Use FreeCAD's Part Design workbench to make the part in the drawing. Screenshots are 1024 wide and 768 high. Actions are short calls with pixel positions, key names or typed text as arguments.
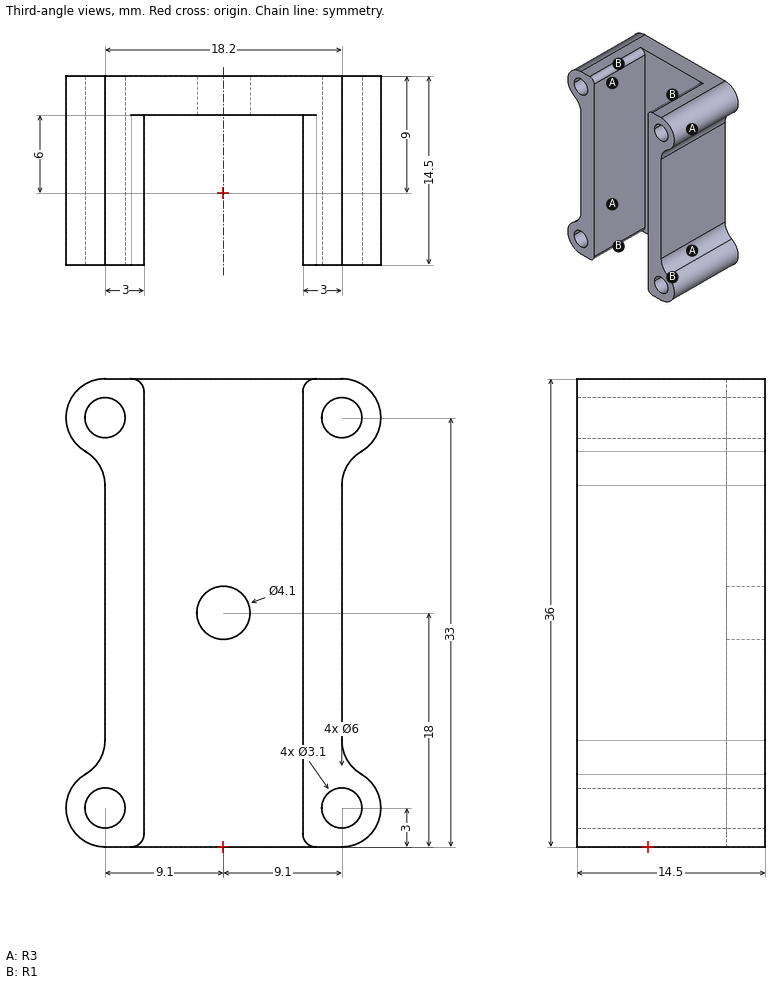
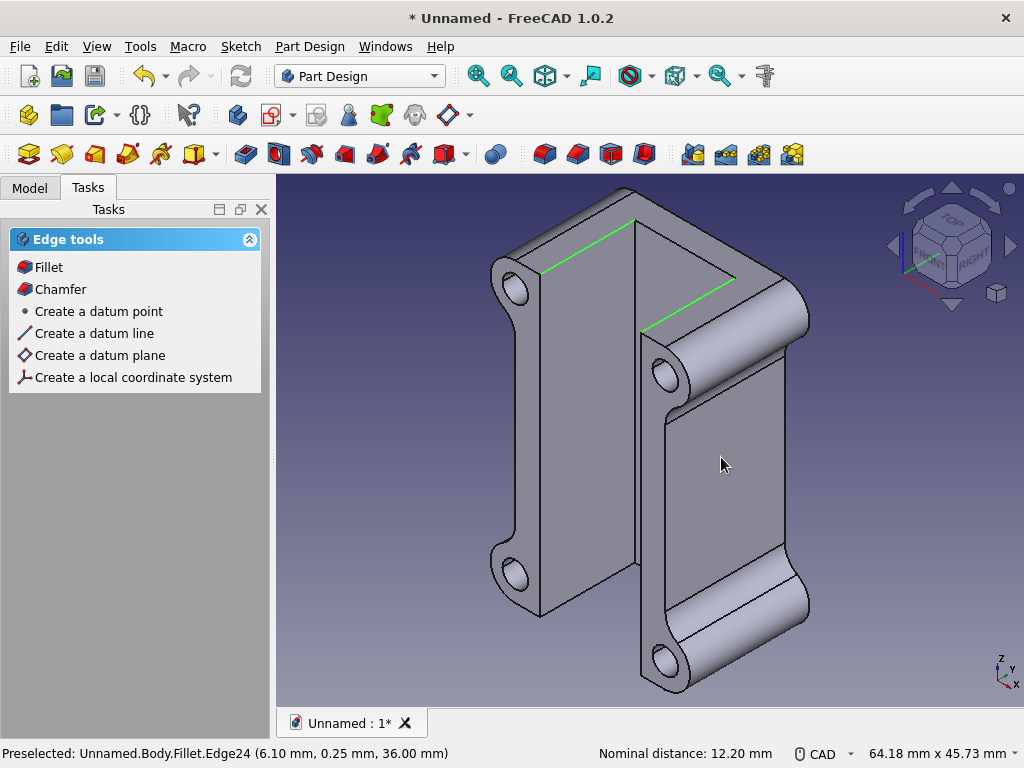
key(1)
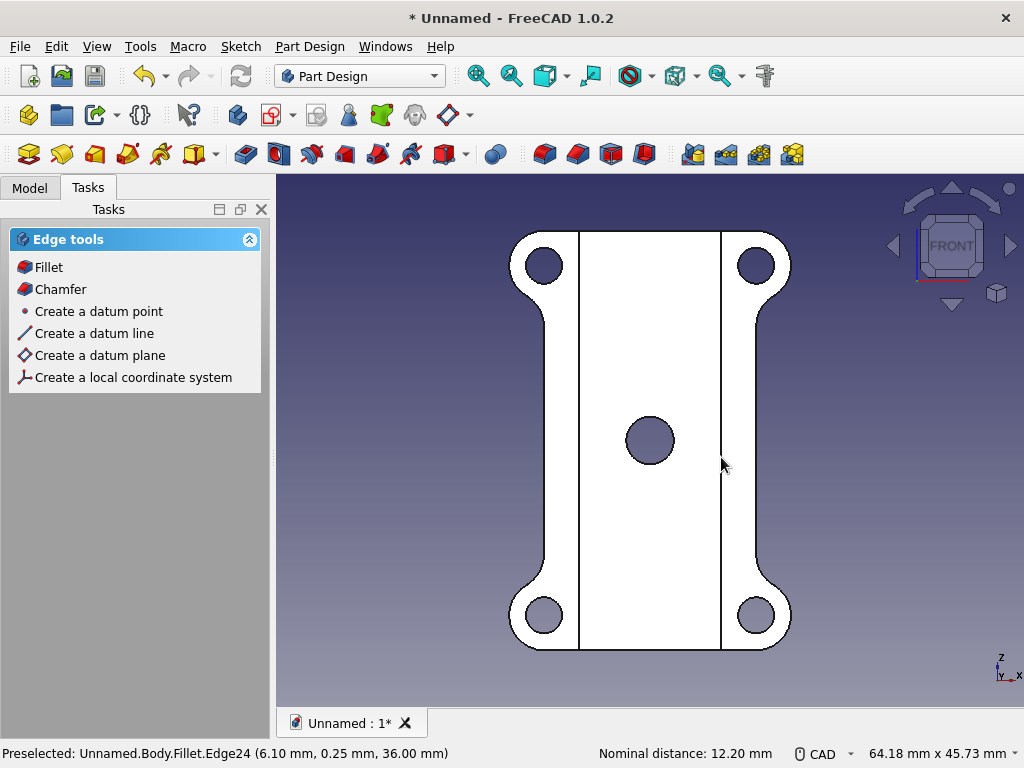
key(3)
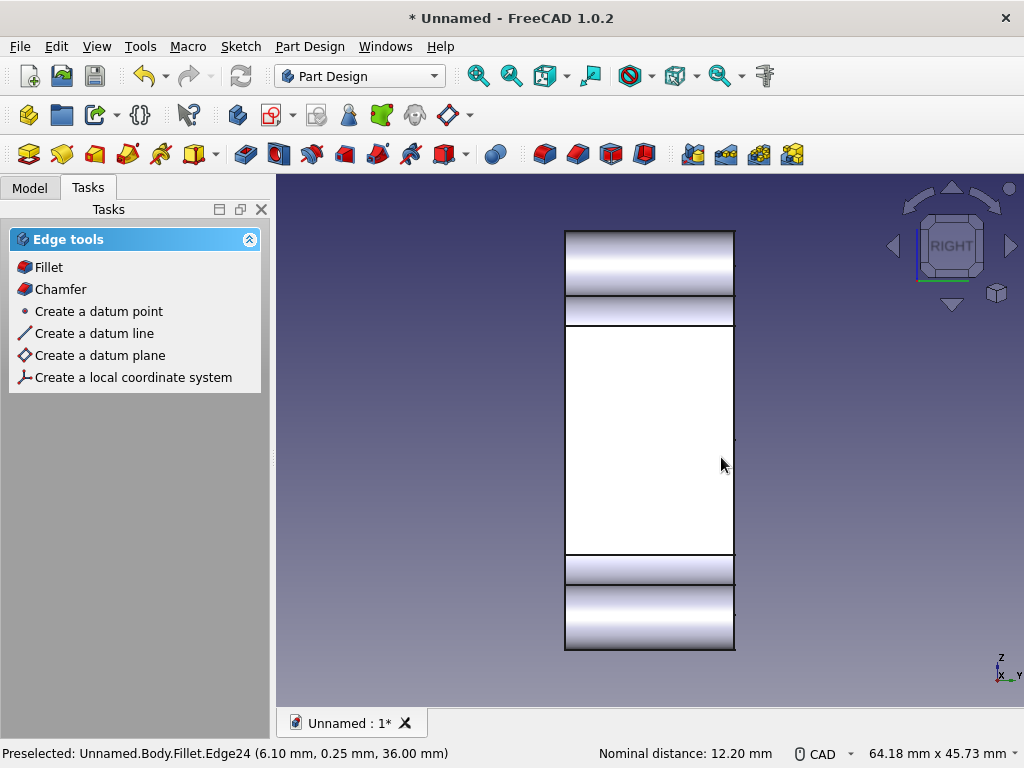
key(5)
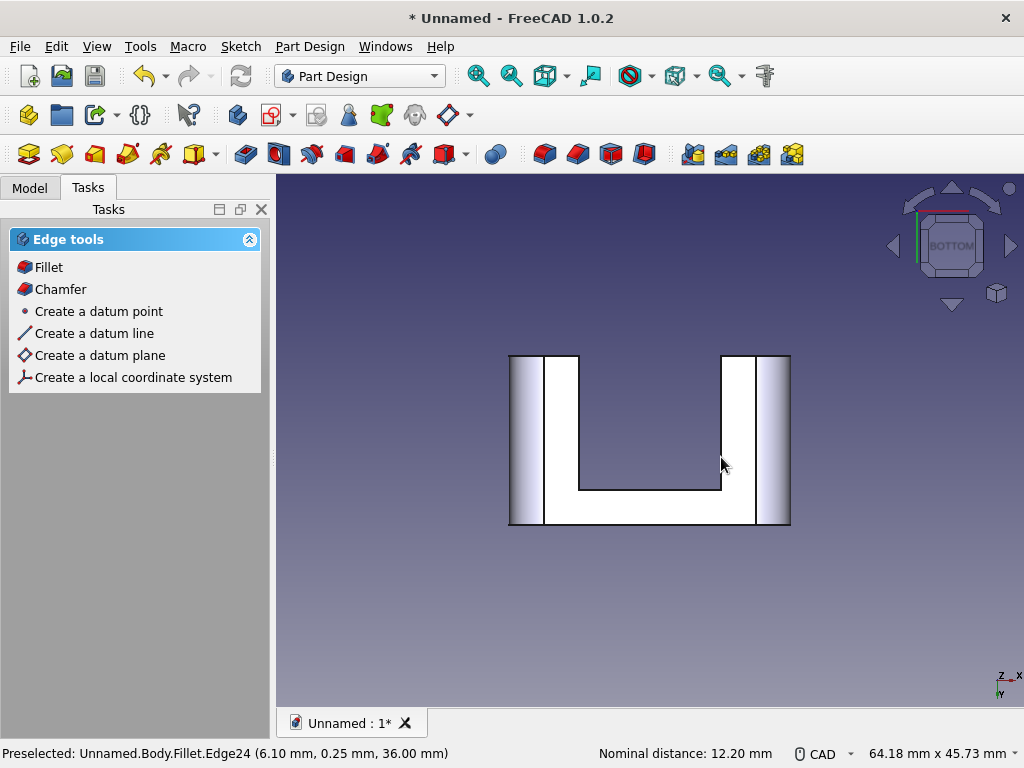
click(479, 76)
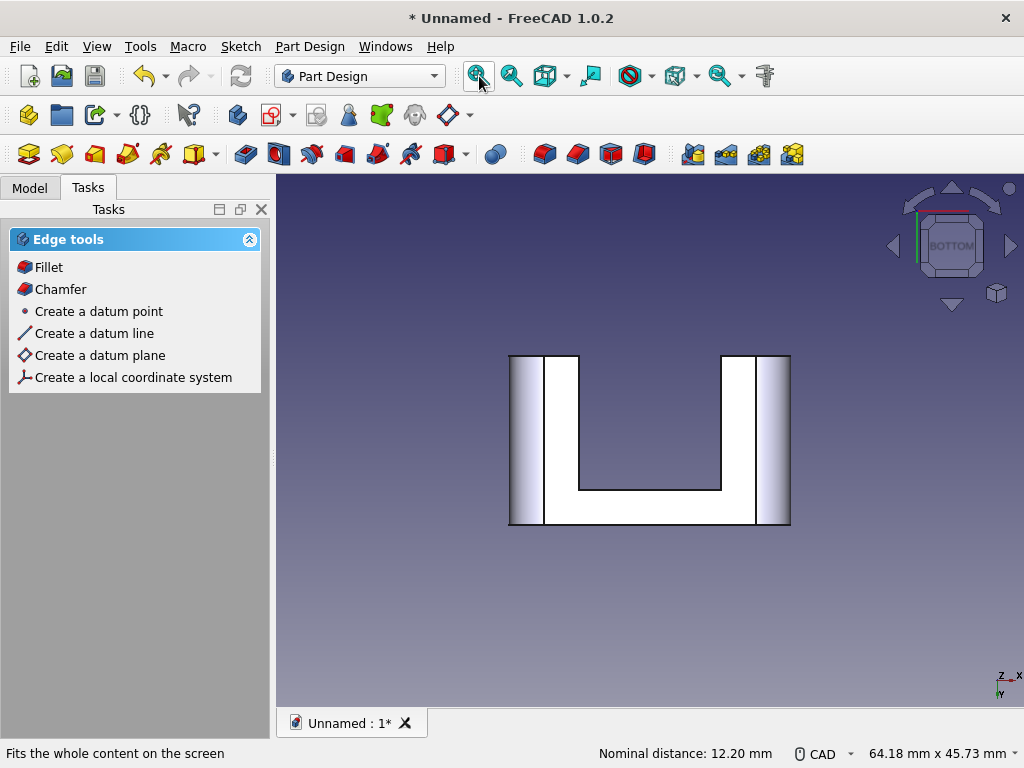
click(721, 422, ctrl)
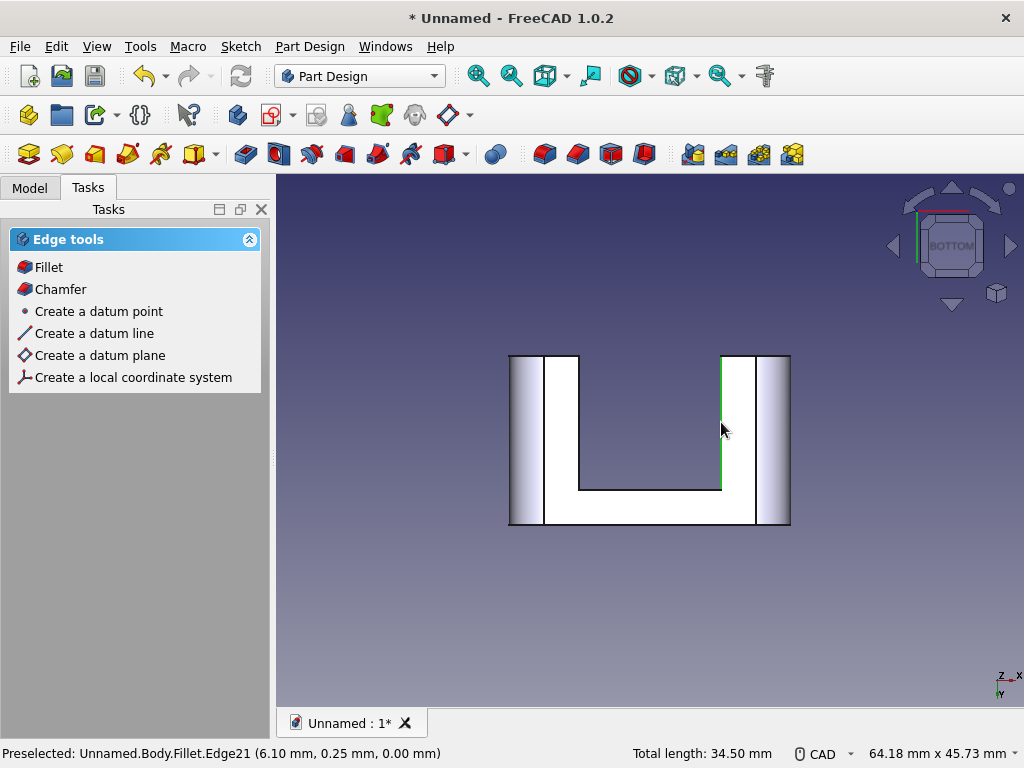
click(579, 422, ctrl)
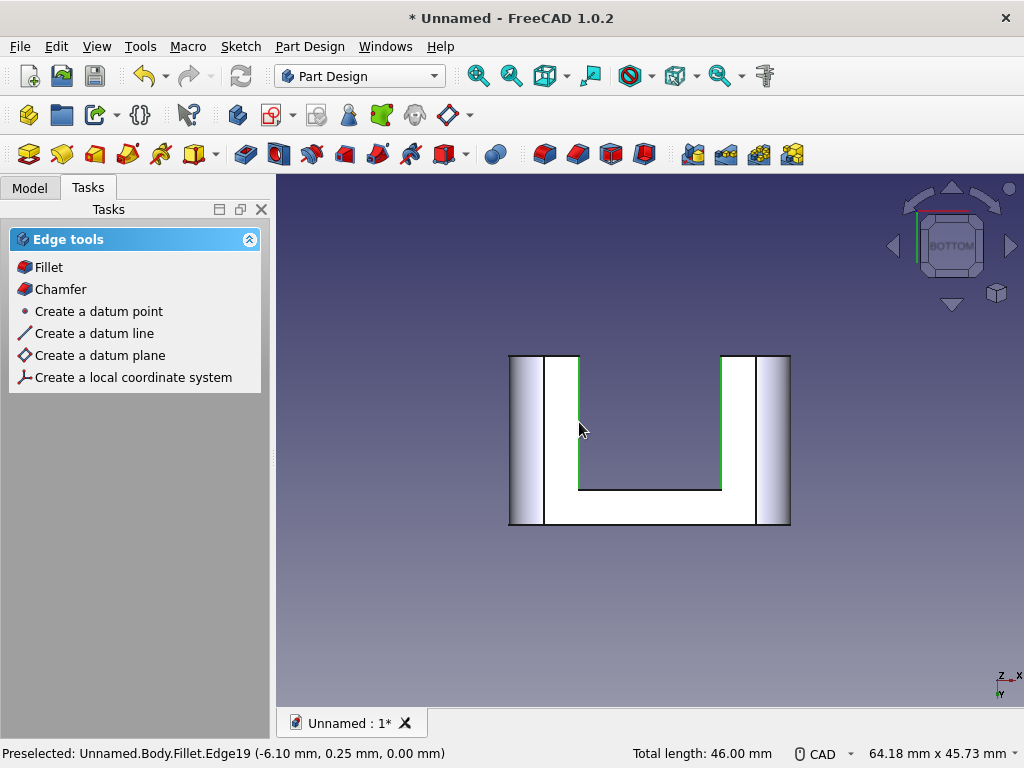
click(545, 154)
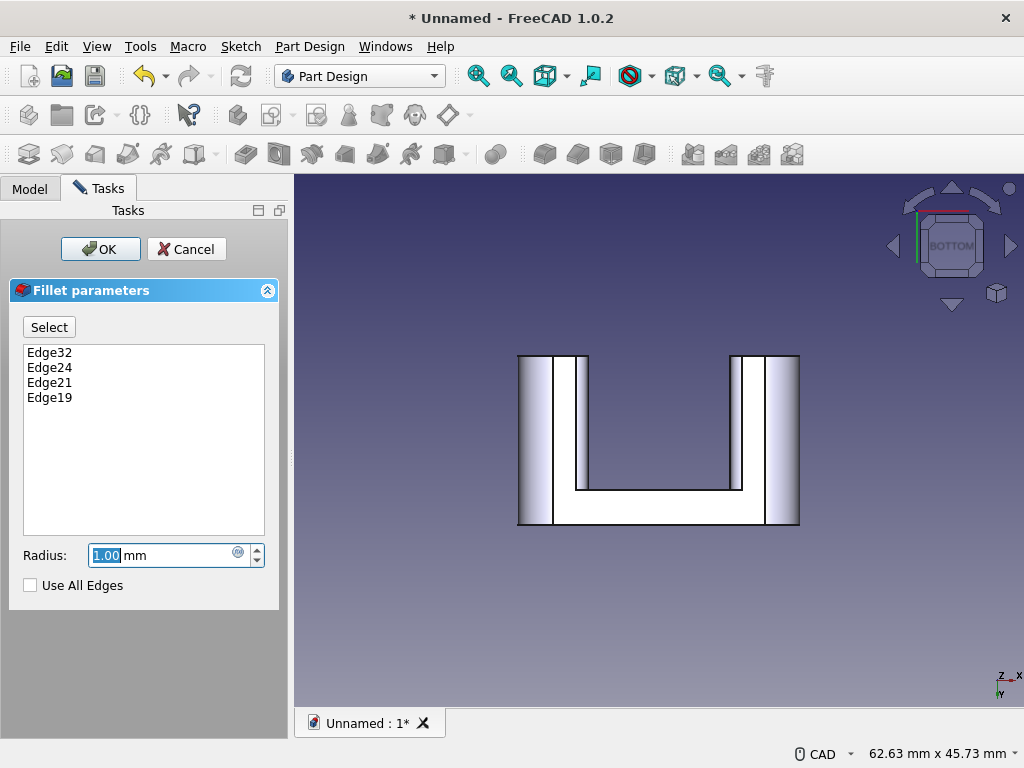
text(1)
key(Tab)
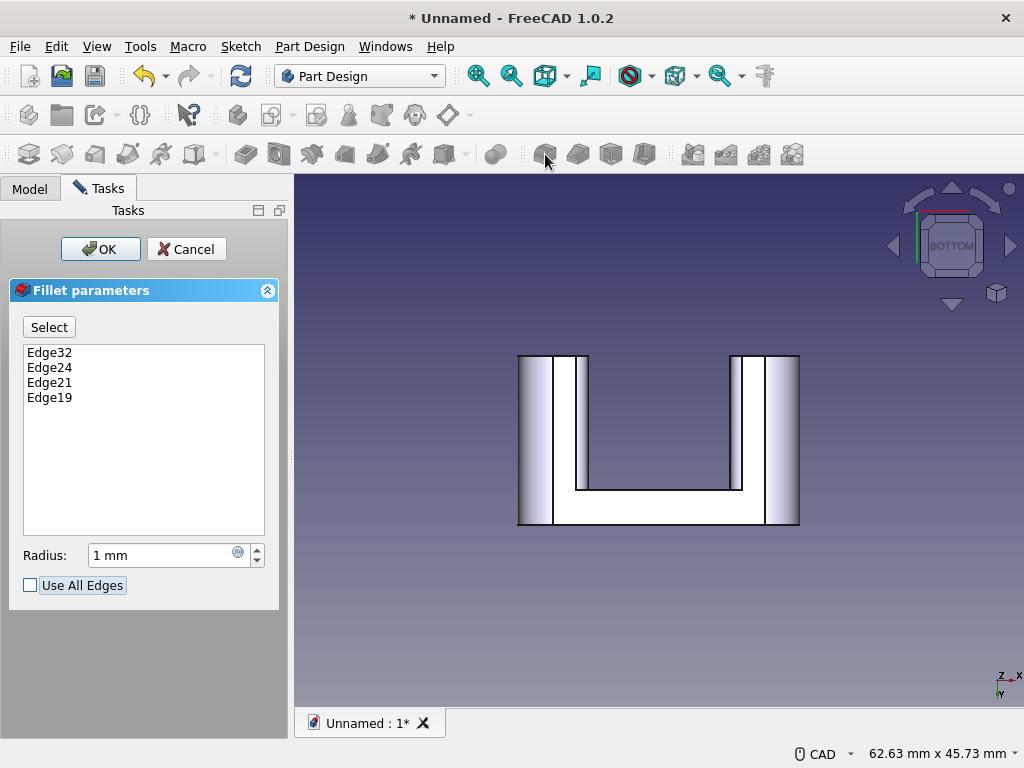
click(101, 249)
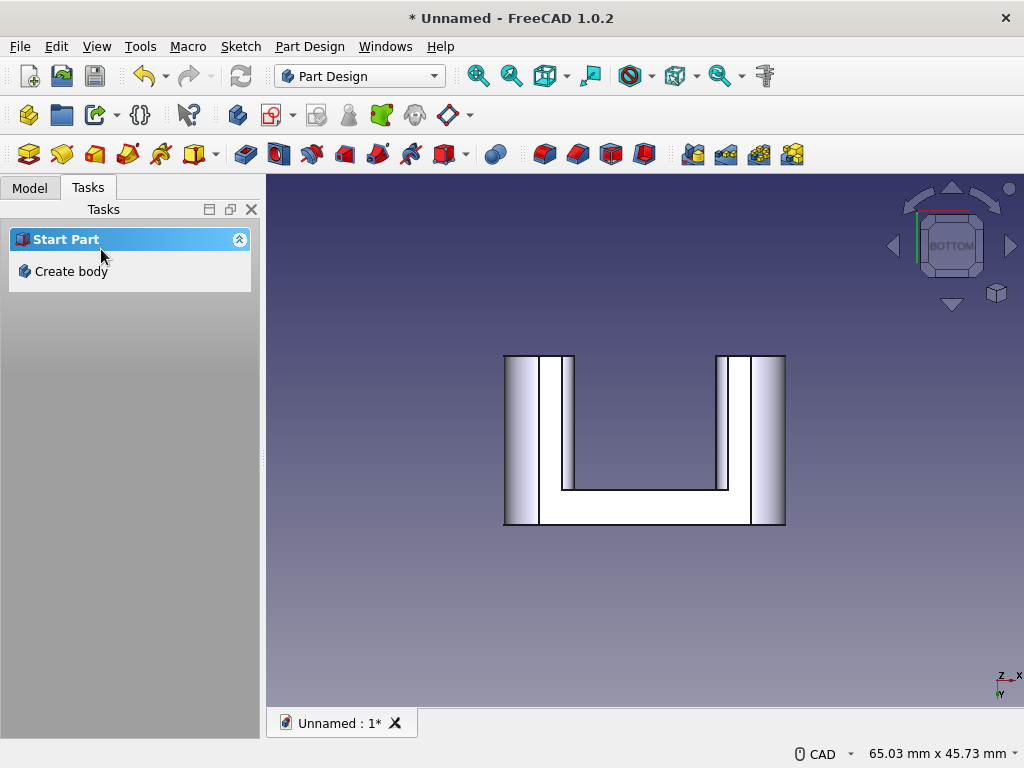
key(0)